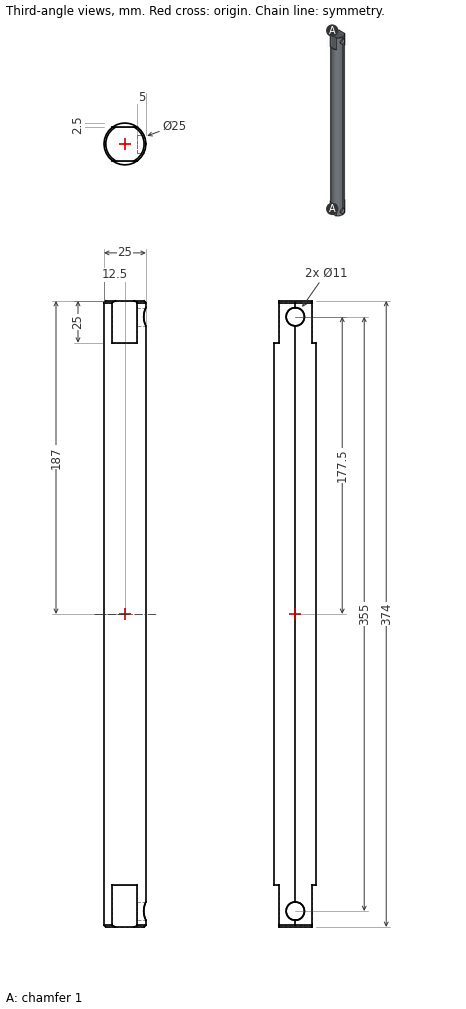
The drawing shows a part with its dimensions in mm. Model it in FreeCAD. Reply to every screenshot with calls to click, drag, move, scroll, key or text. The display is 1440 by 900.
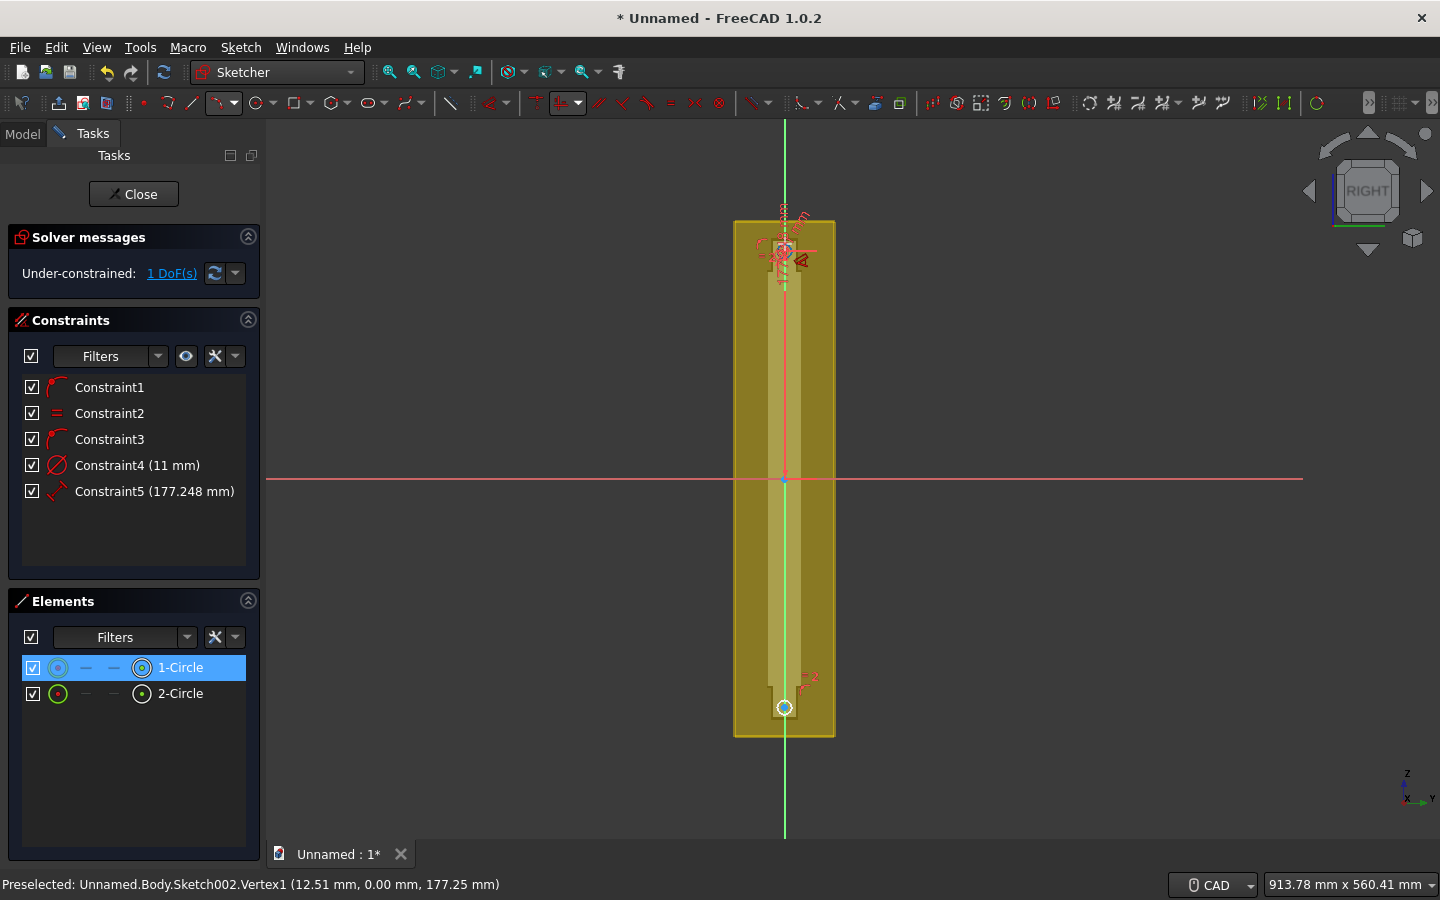
click(785, 708)
click(819, 375)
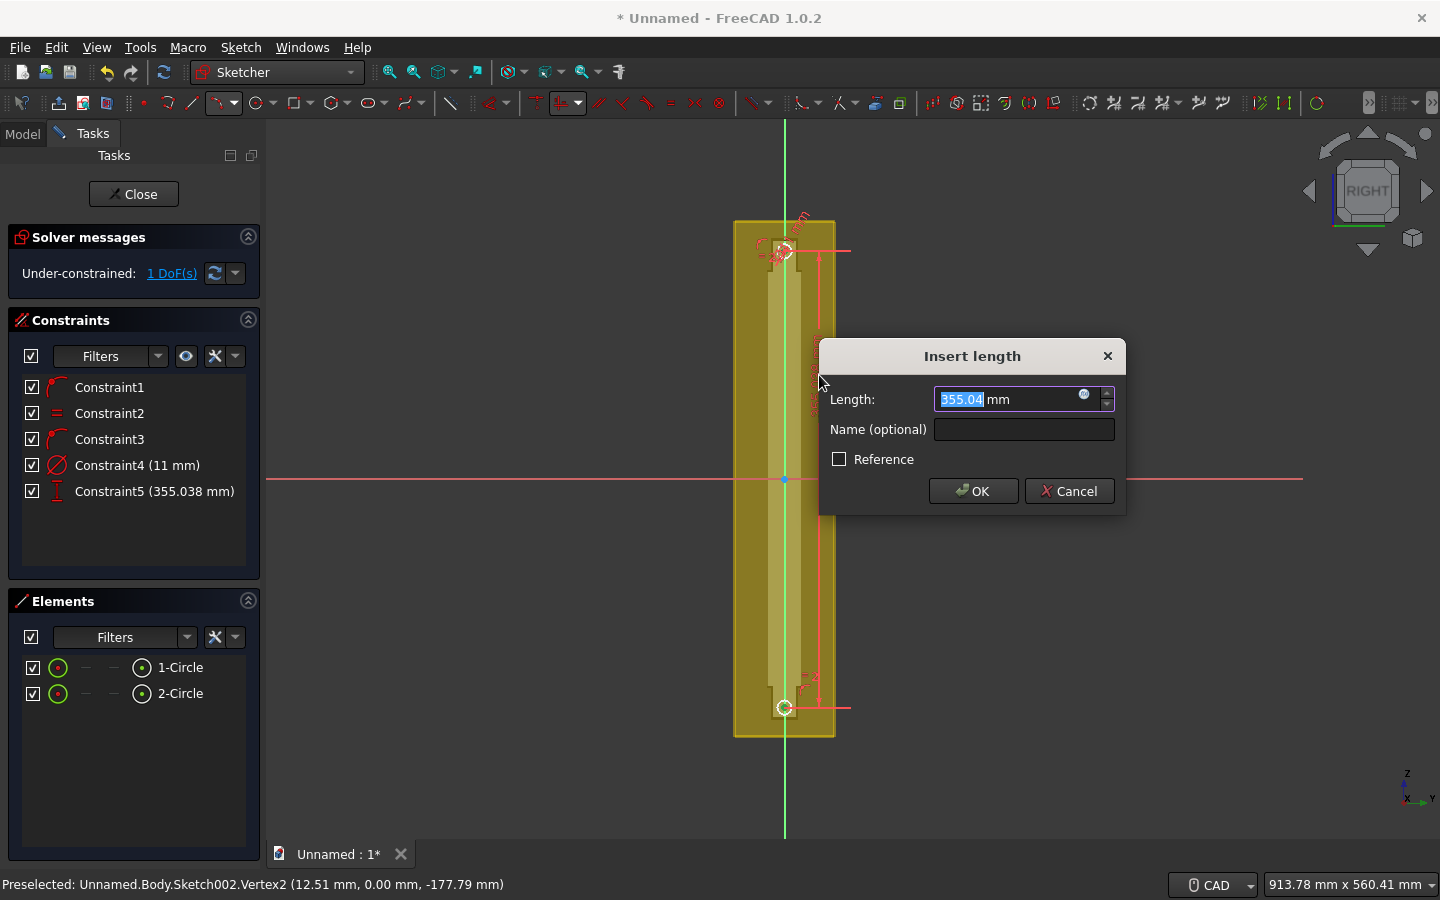
text(355)
key(Return)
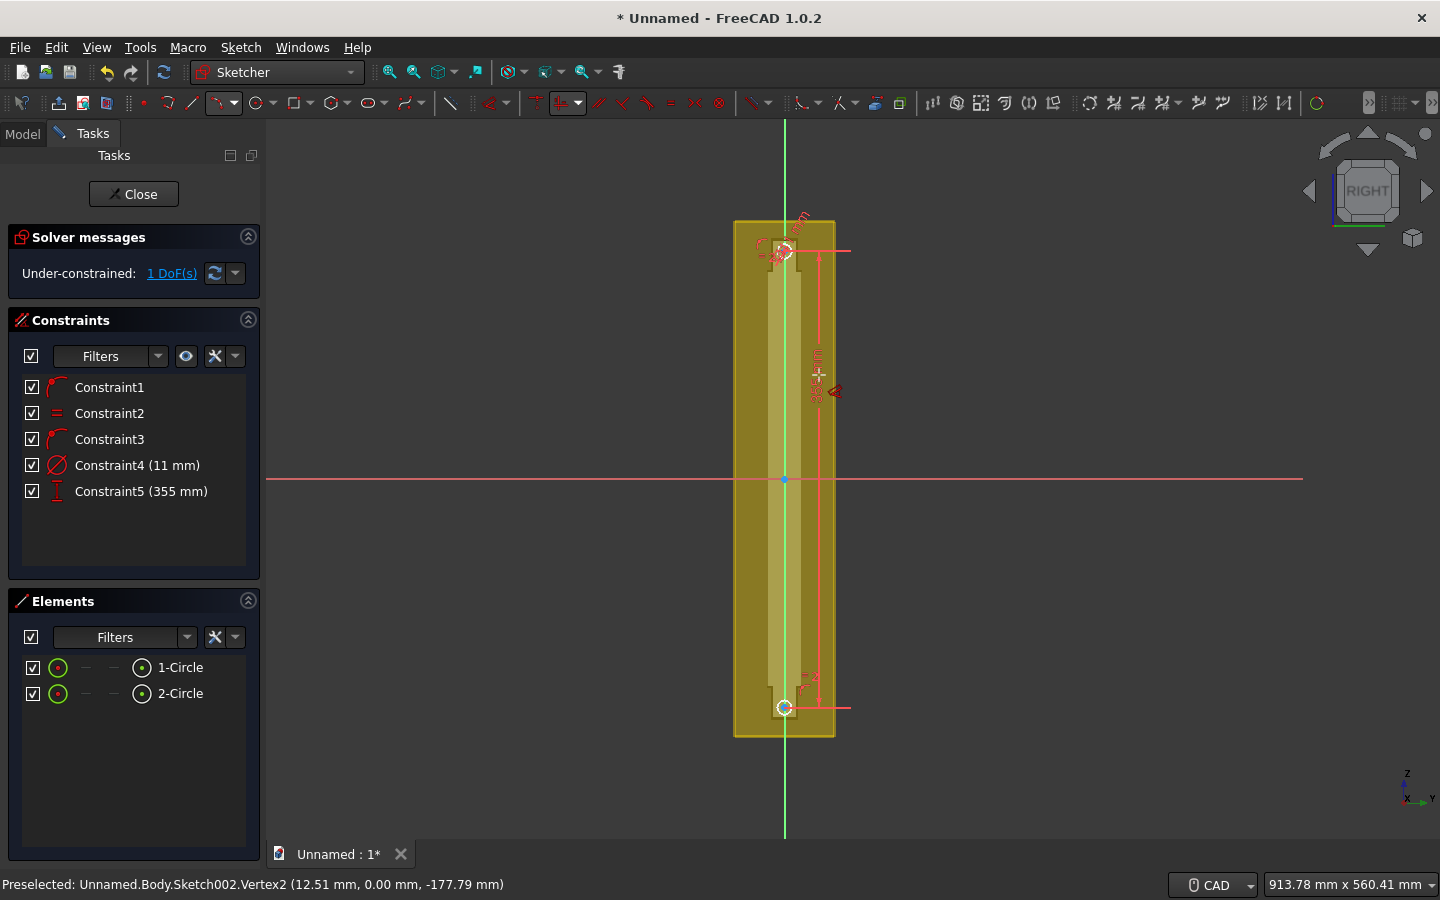
click(785, 251)
click(819, 313)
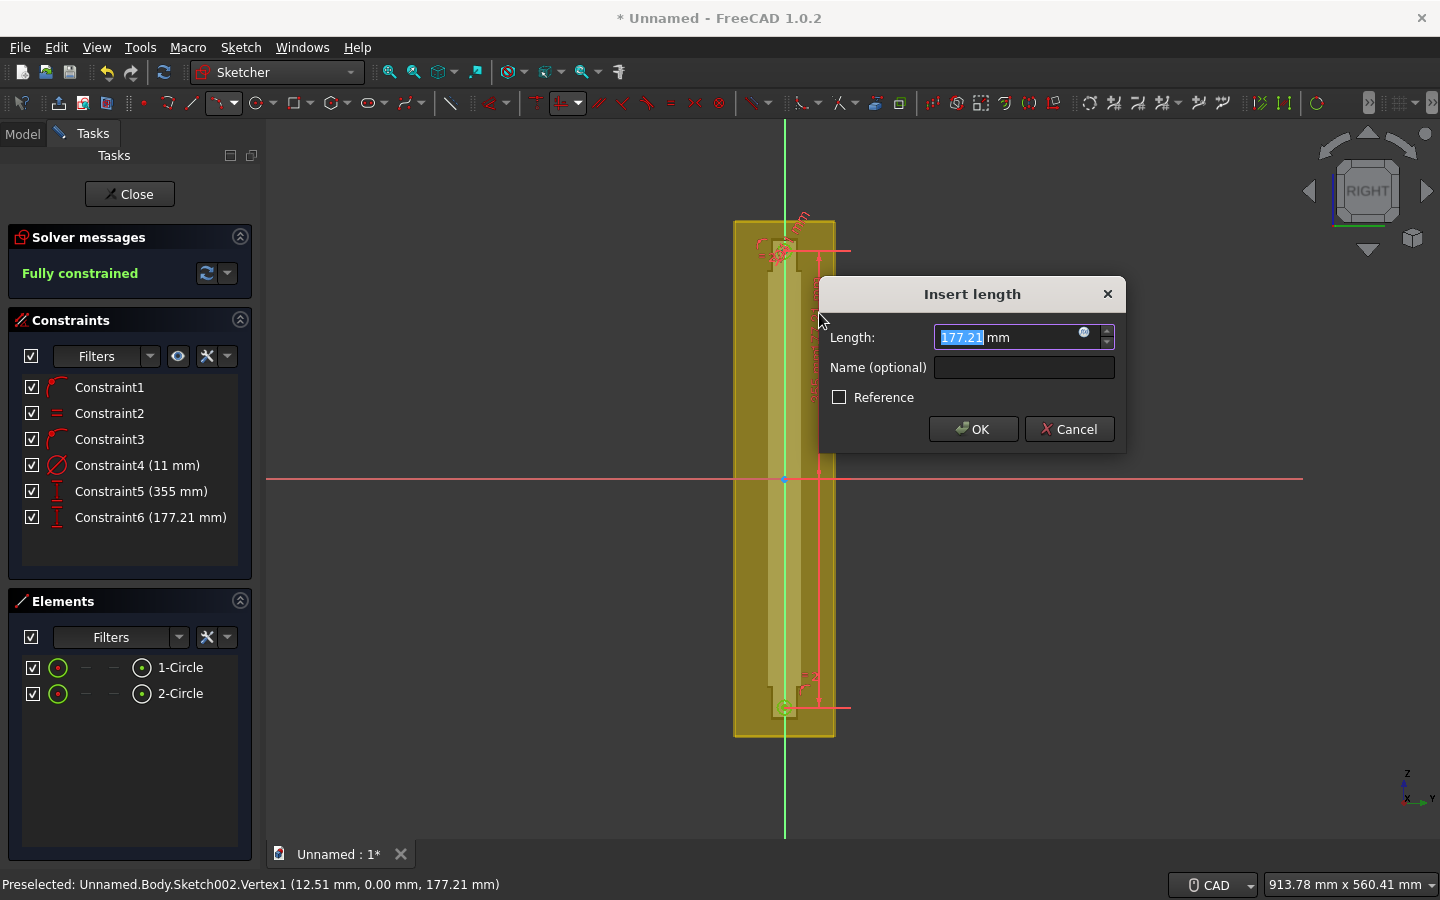
text(177.5)
key(Return)
key(Escape)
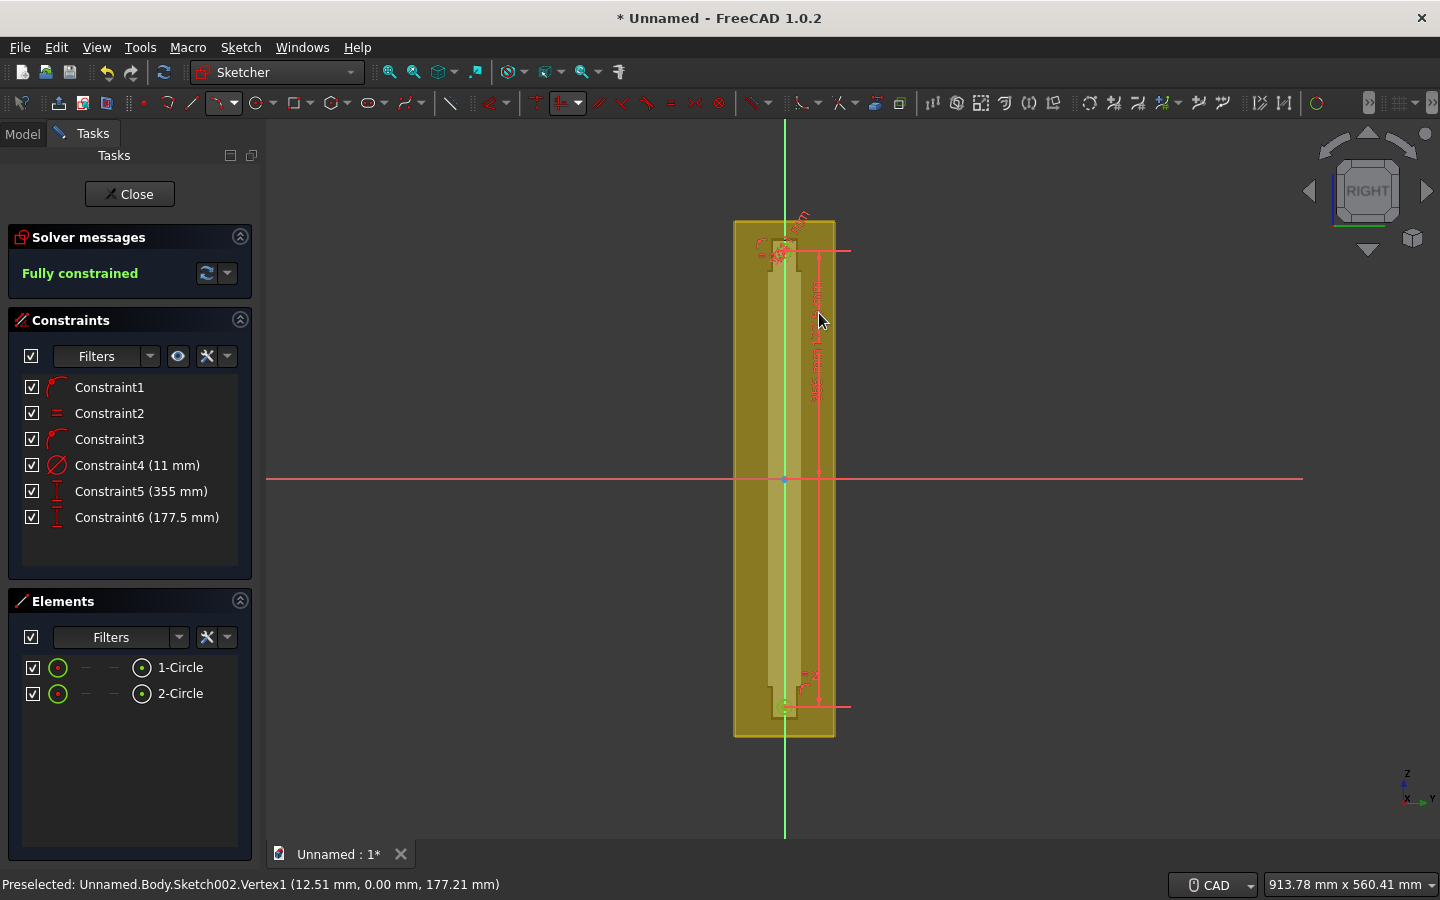
click(130, 194)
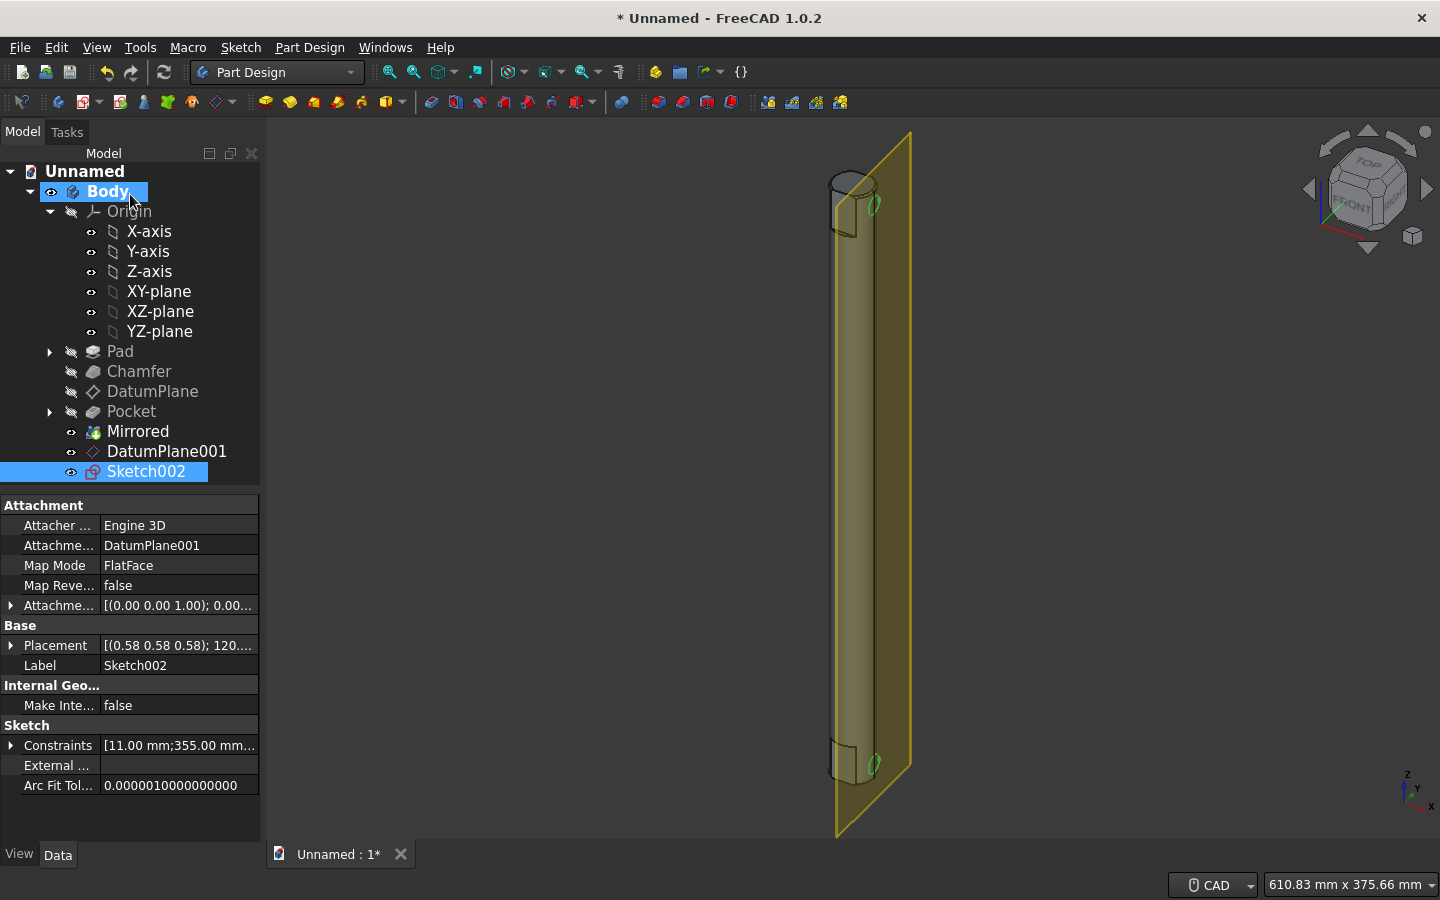
click(432, 102)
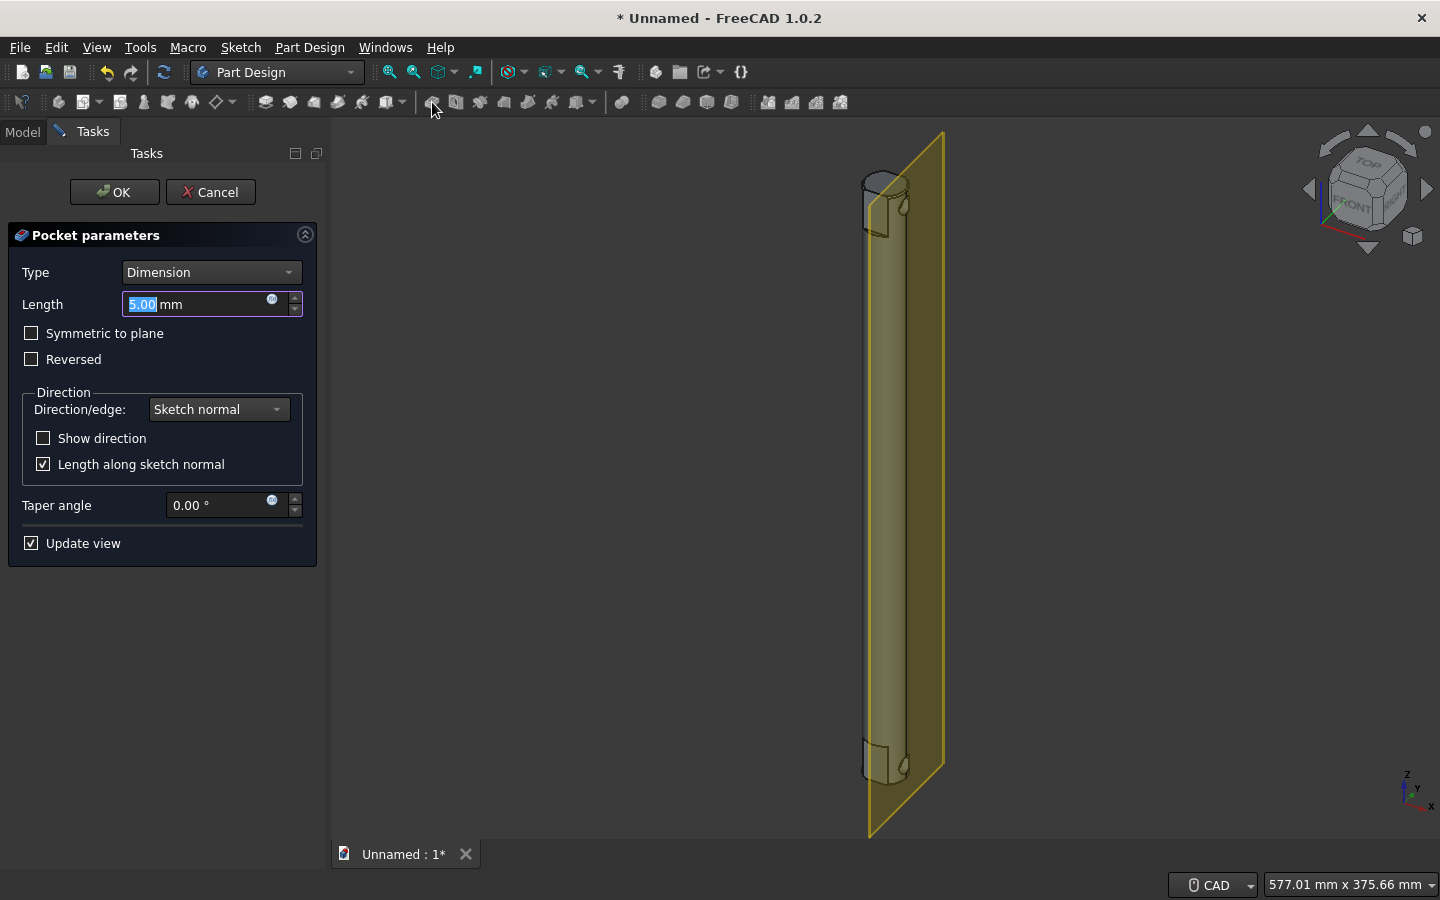
text(5)
key(Tab)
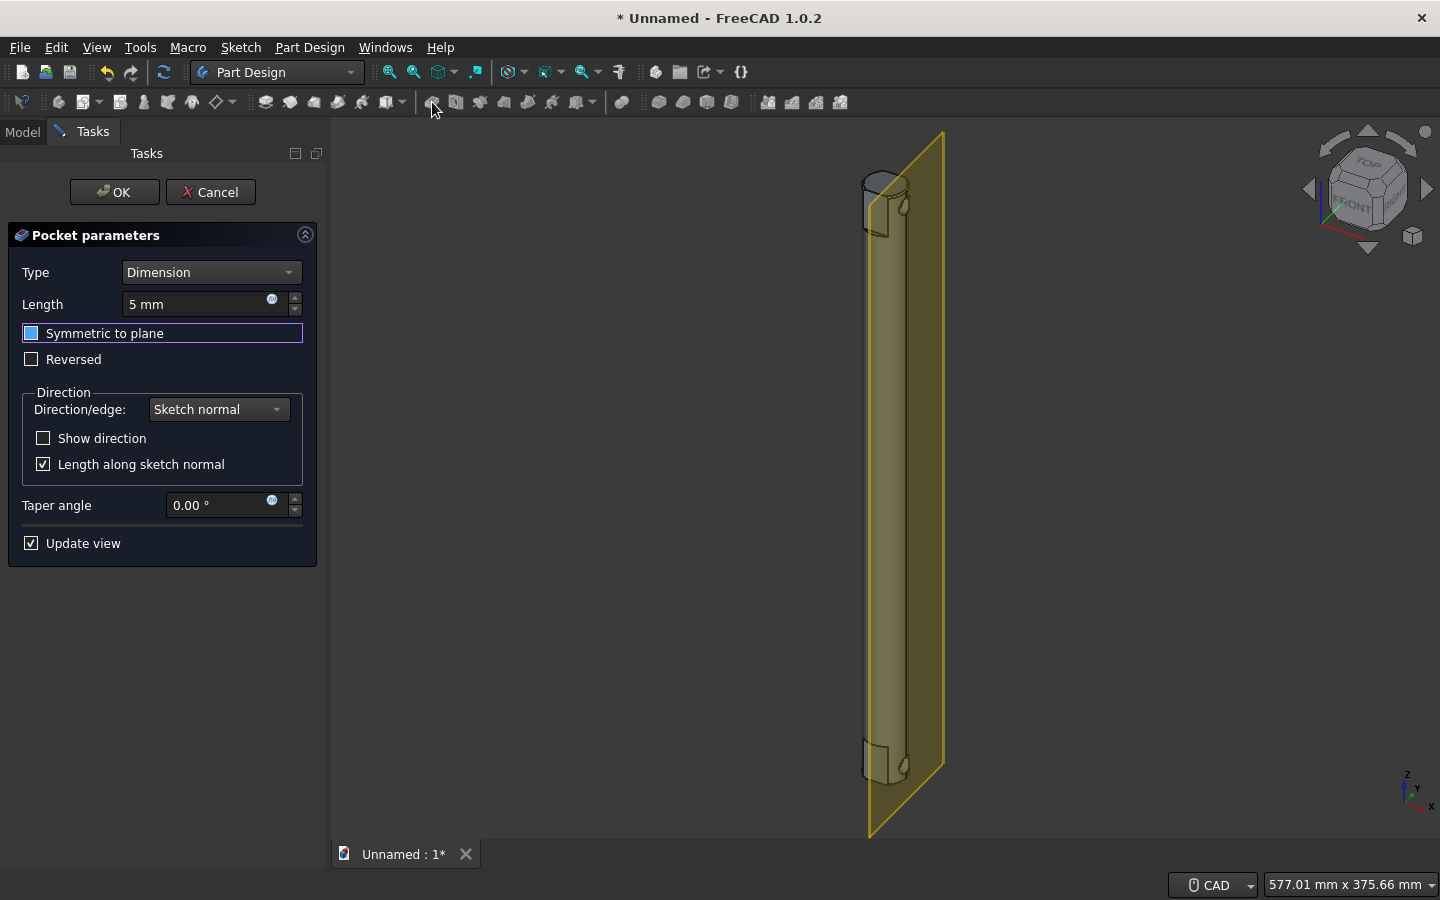
click(115, 192)